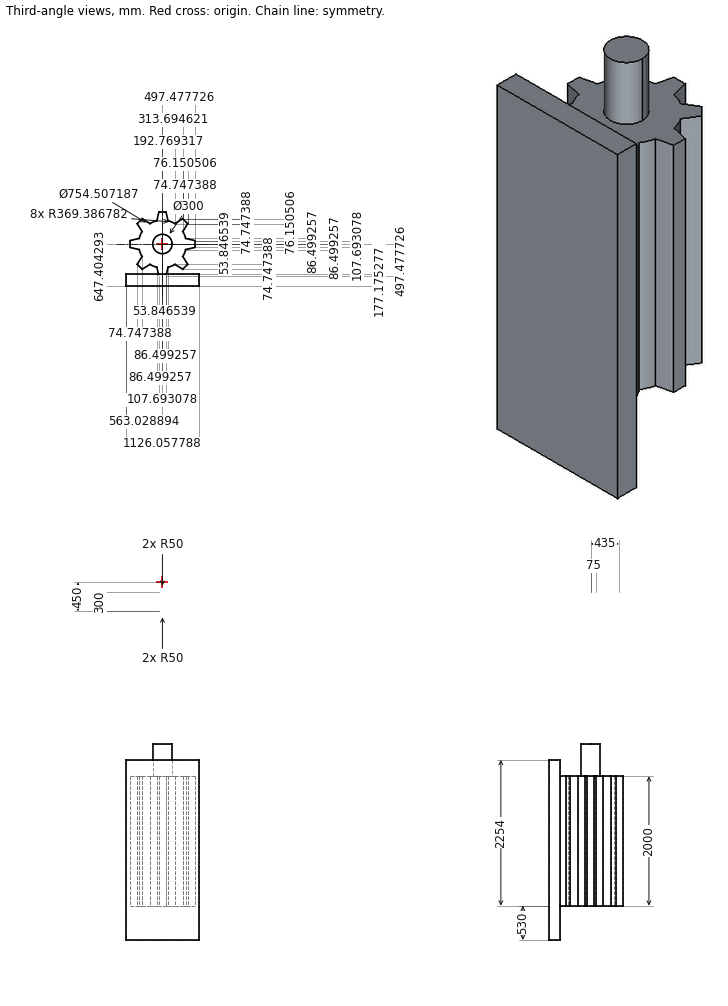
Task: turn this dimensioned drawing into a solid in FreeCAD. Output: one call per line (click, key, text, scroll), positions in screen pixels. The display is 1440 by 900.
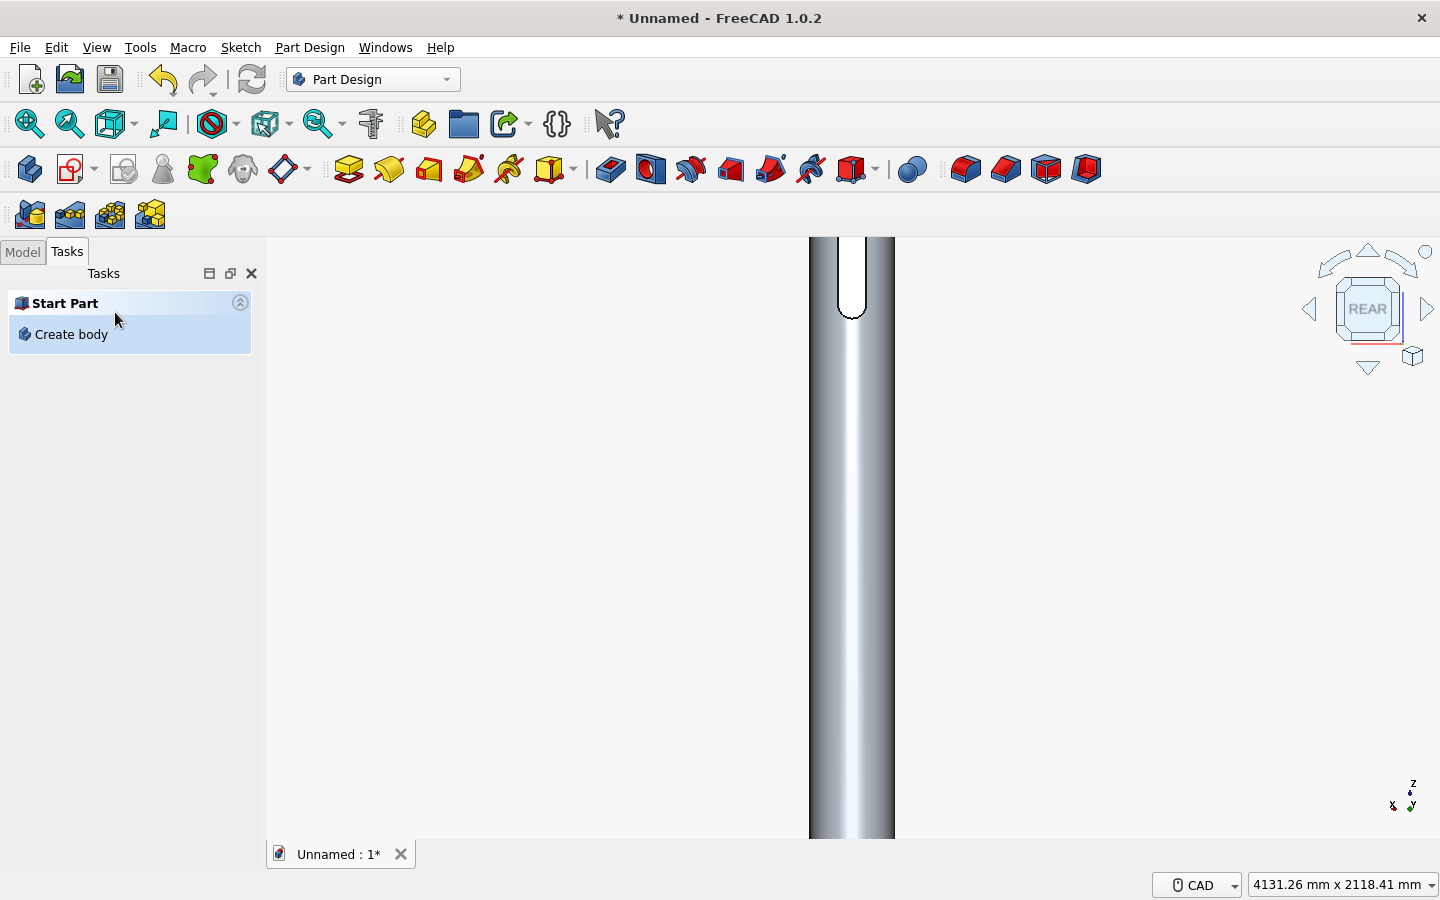
click(30, 124)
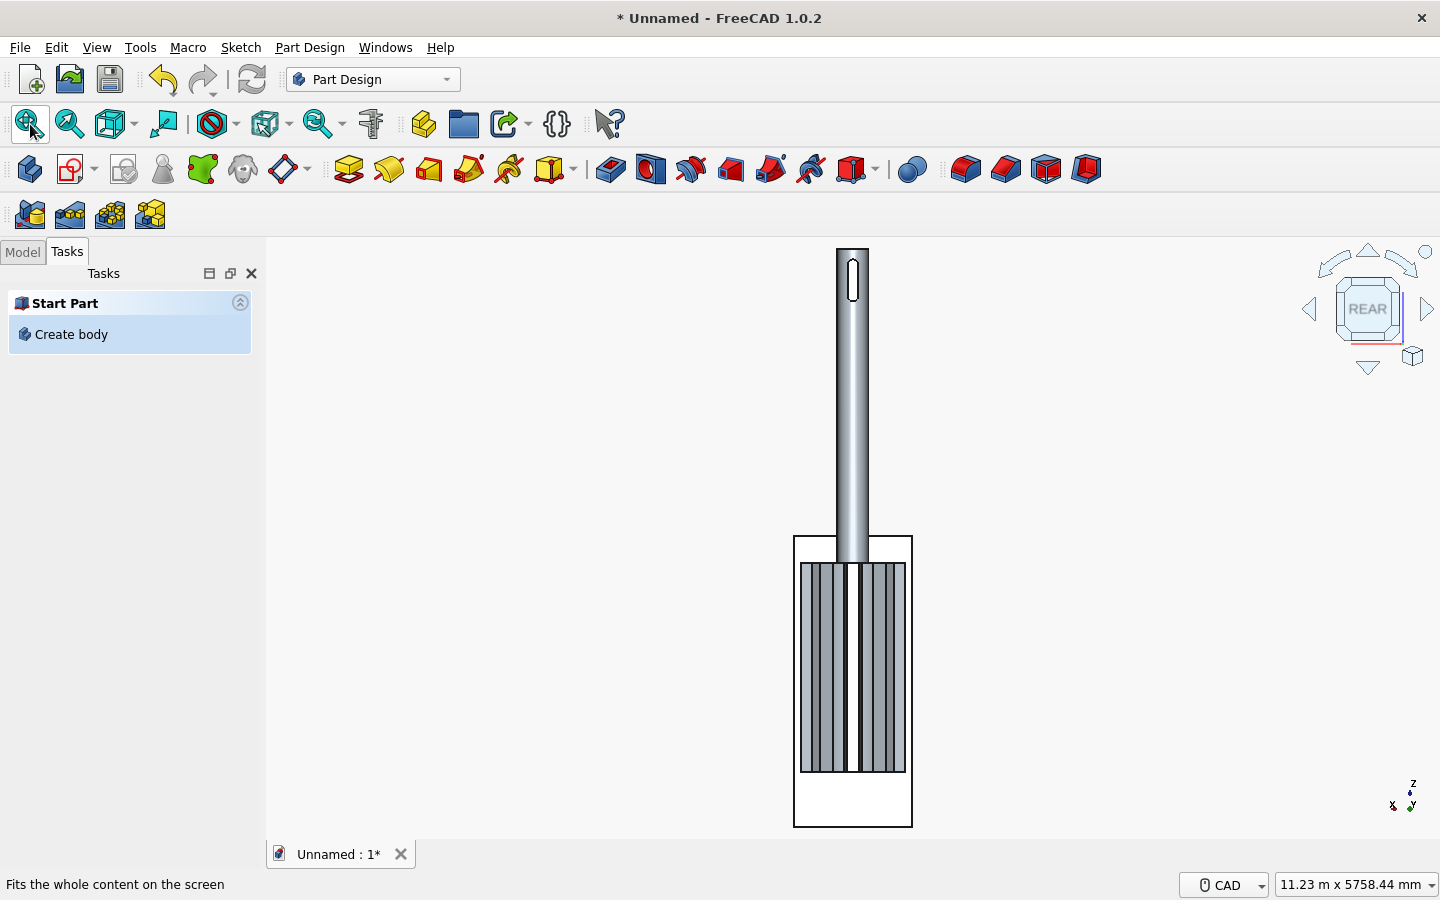
click(70, 170)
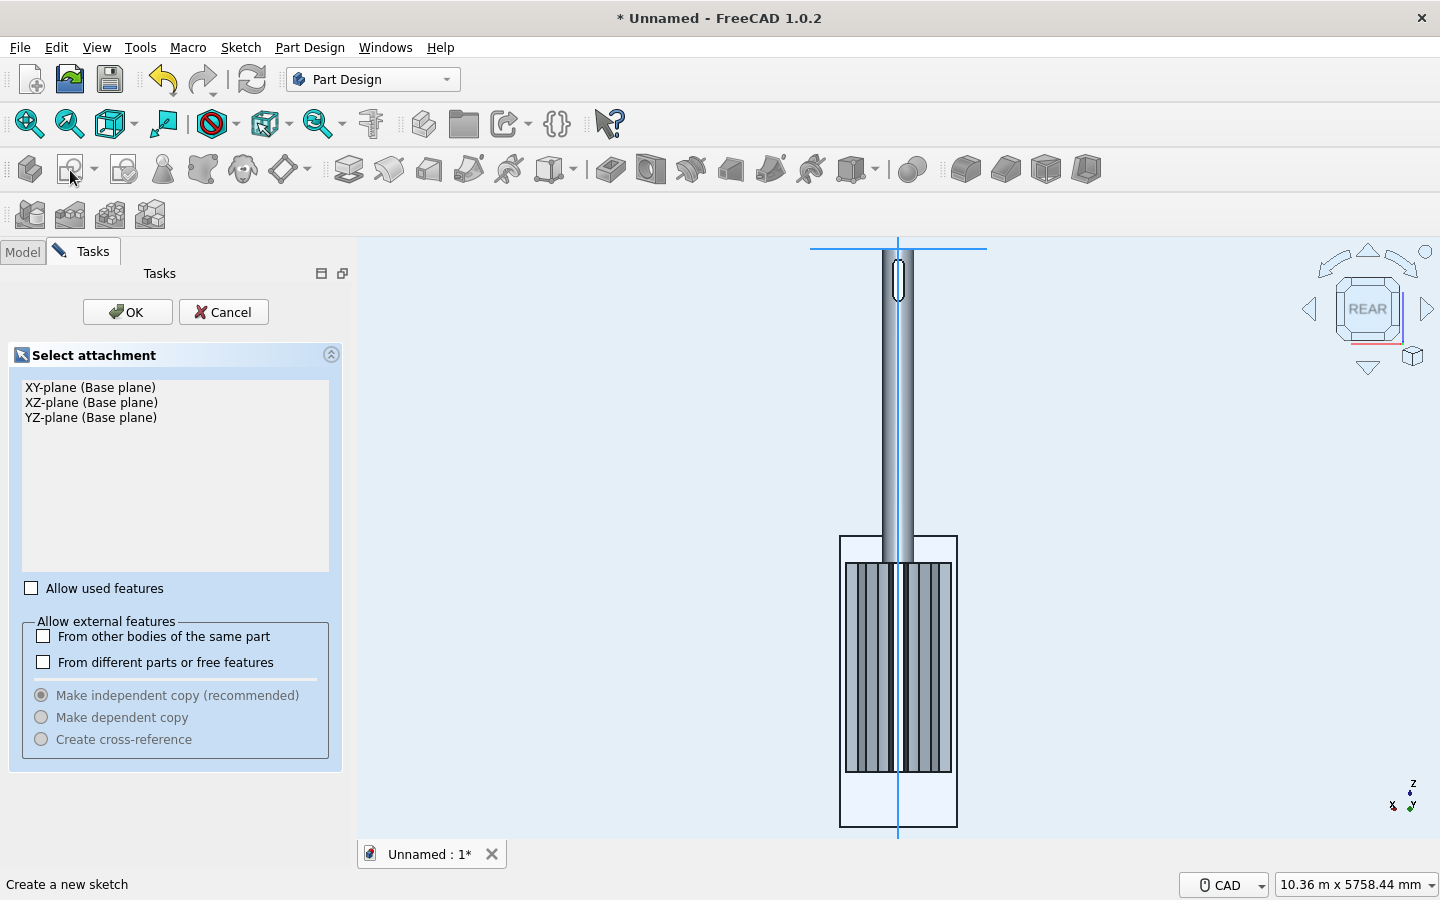
click(82, 388)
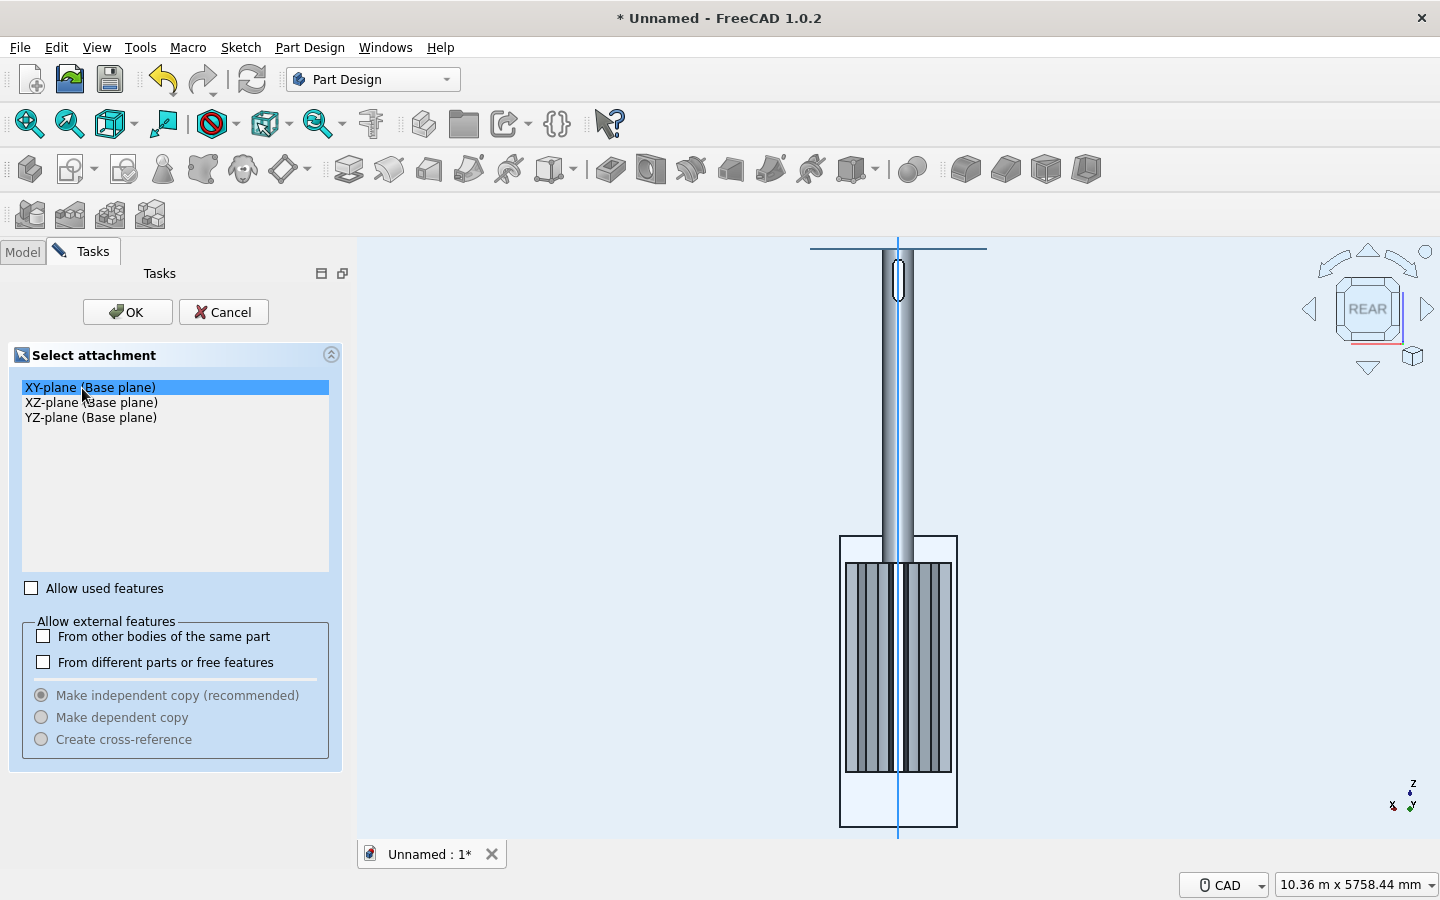
click(128, 312)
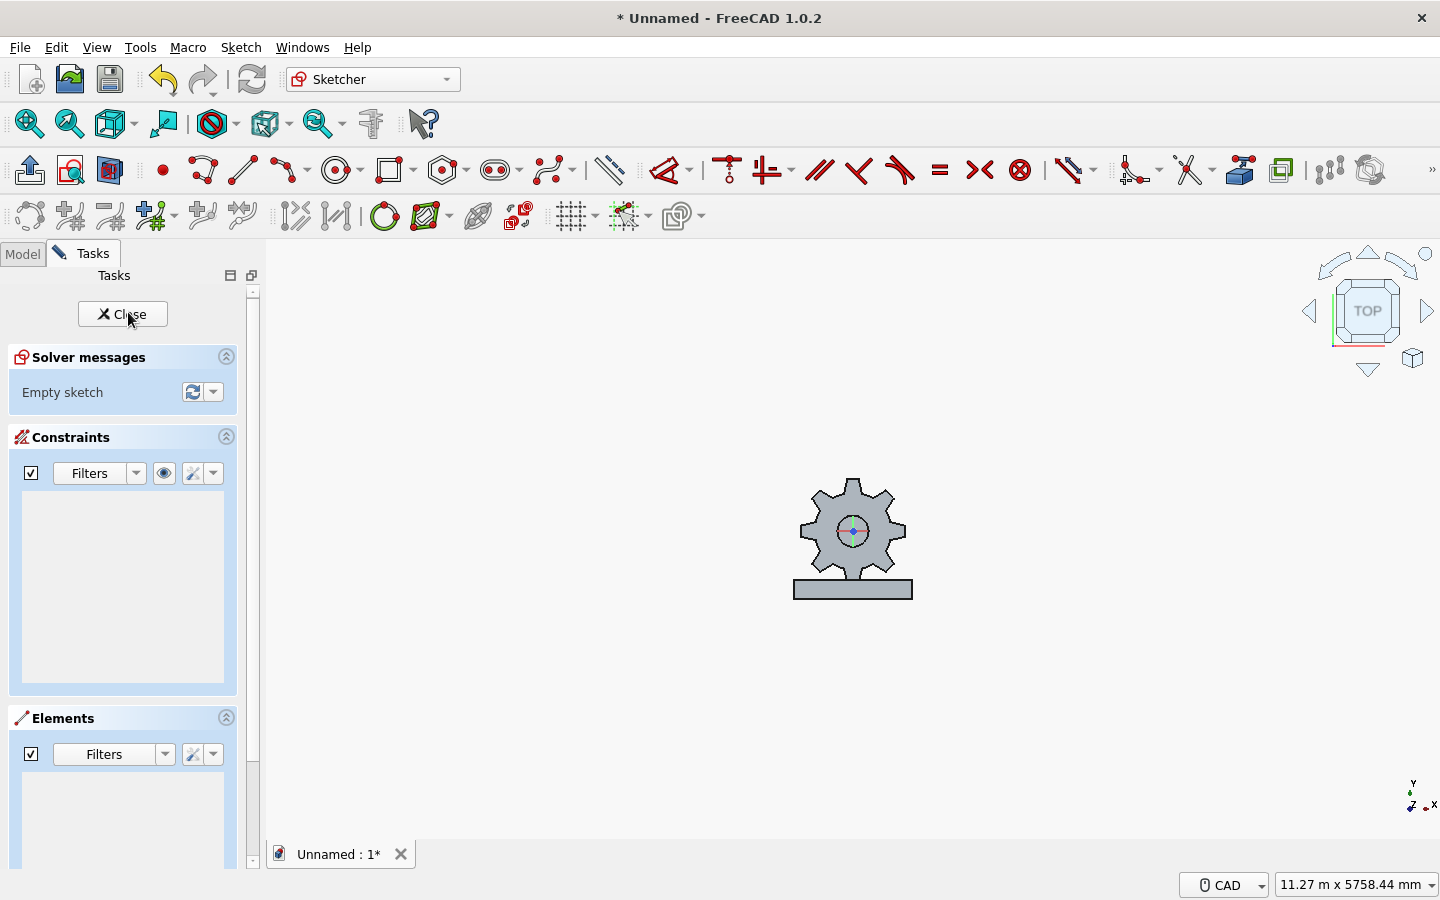
scroll(870, 529, up, 8)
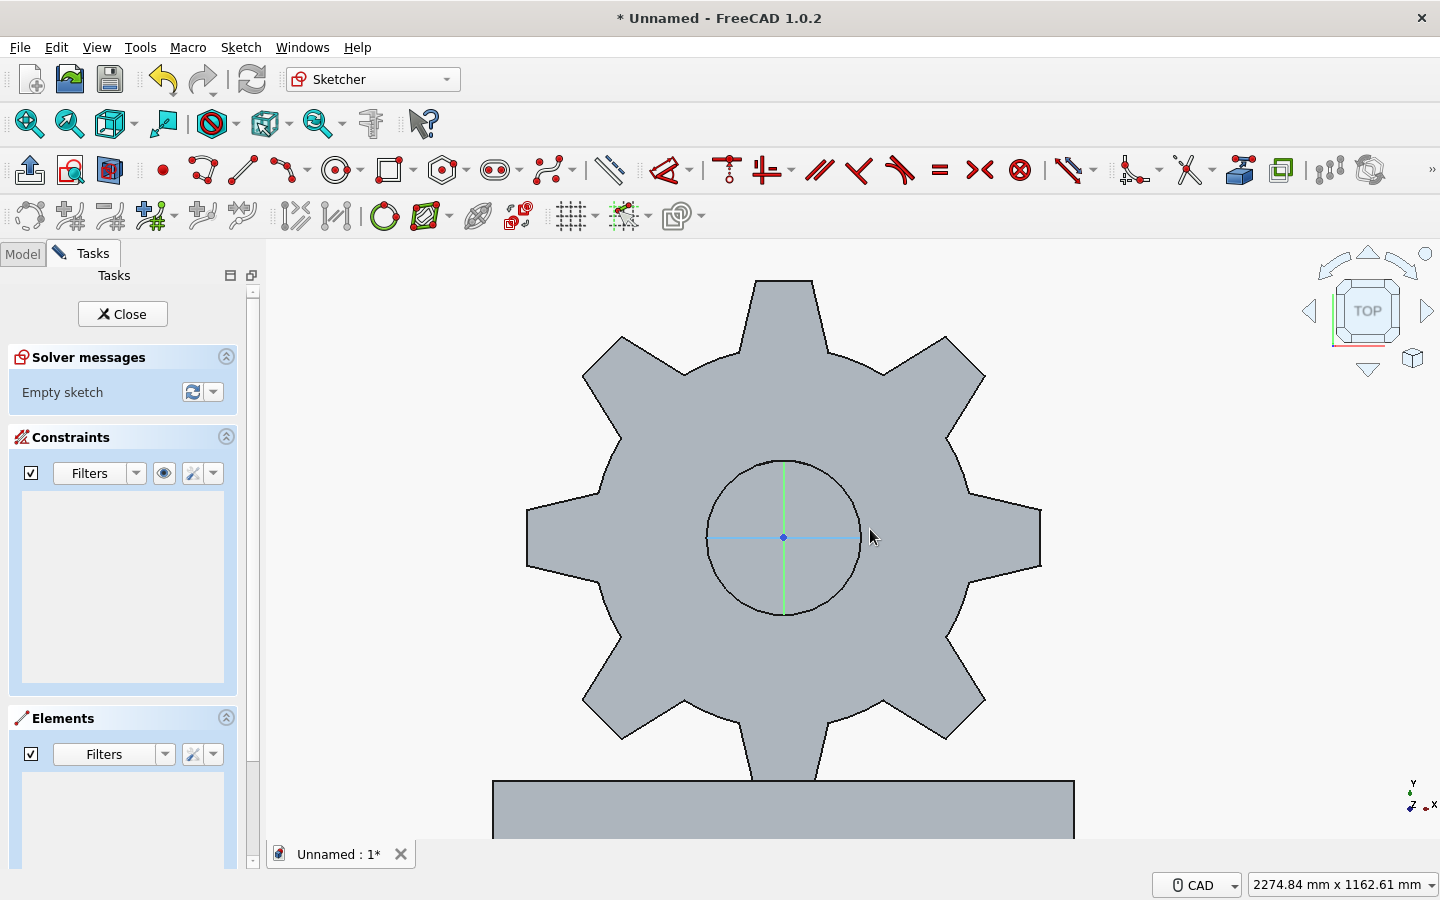
click(336, 170)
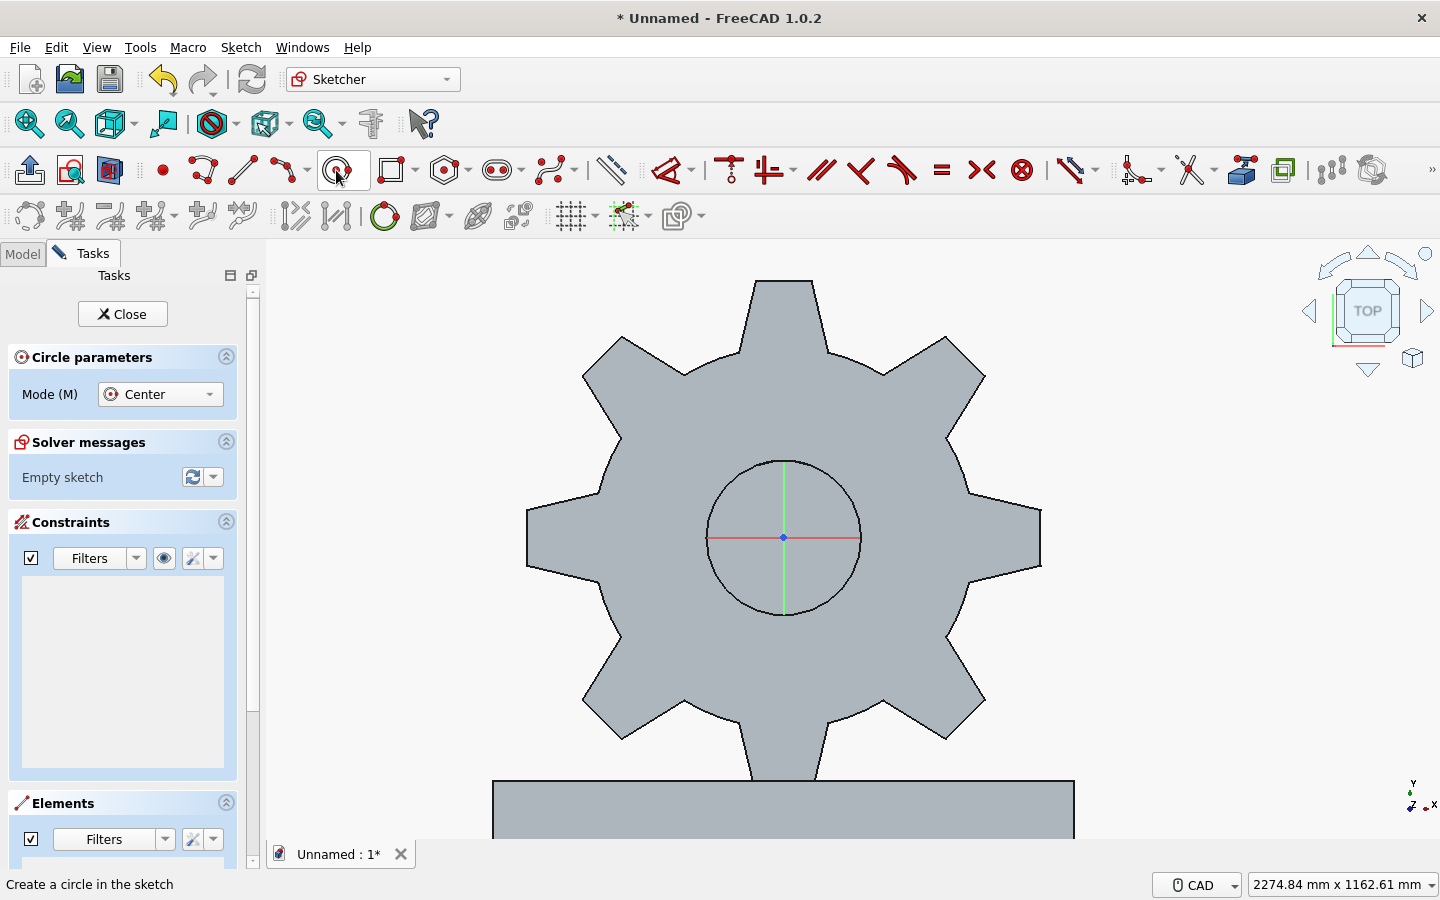
click(784, 538)
move(921, 400)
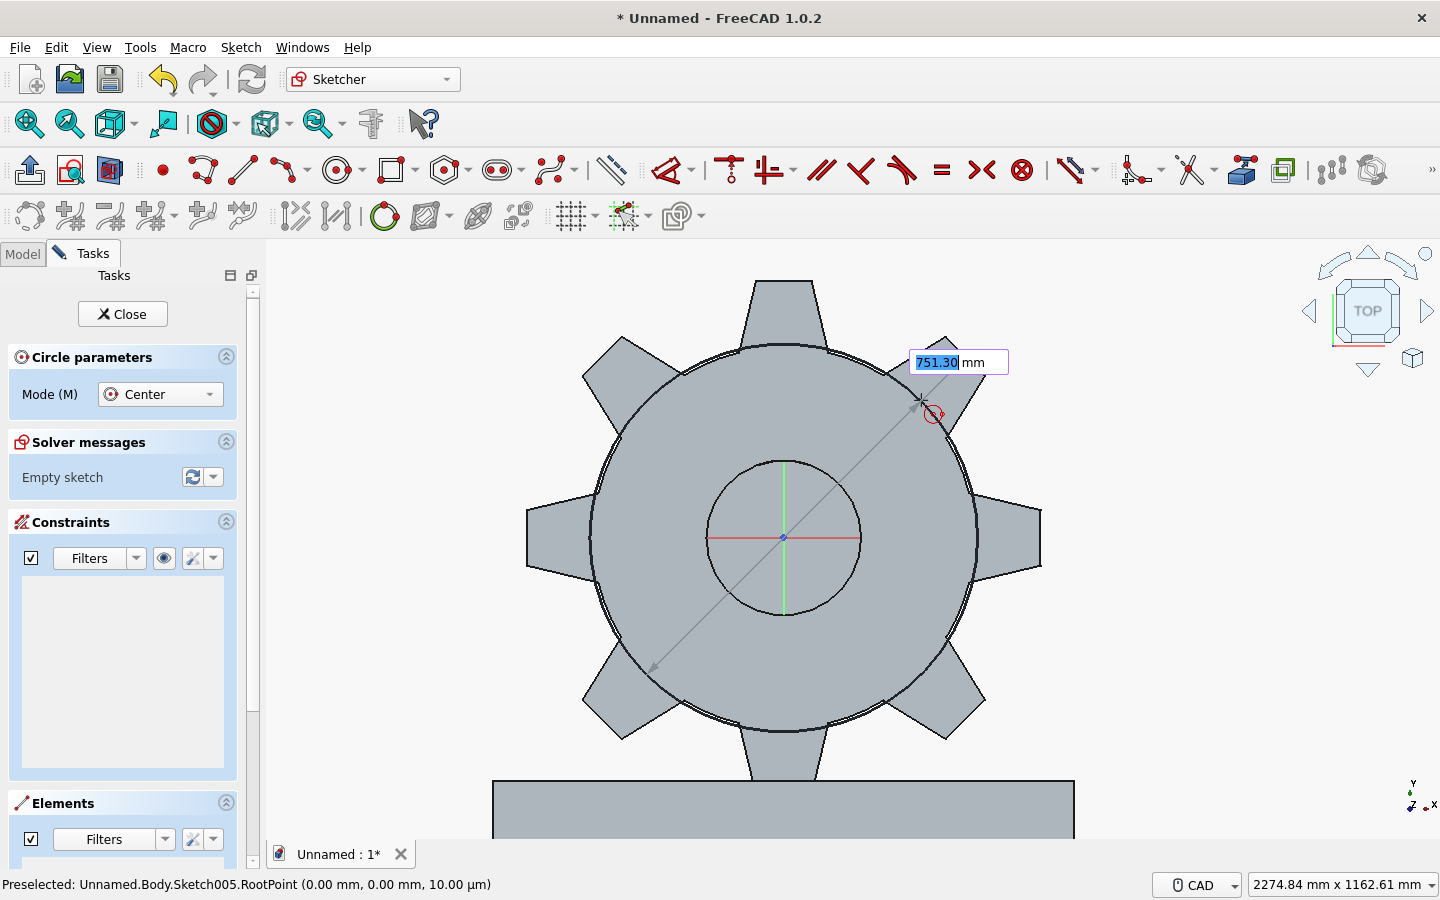
text(754.507187)
key(Return)
key(Escape)